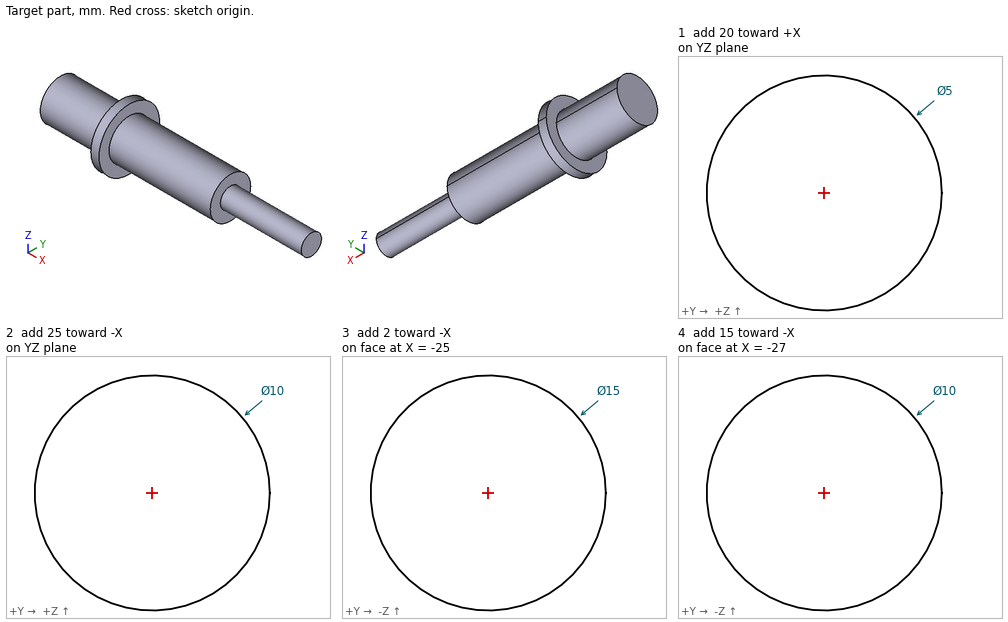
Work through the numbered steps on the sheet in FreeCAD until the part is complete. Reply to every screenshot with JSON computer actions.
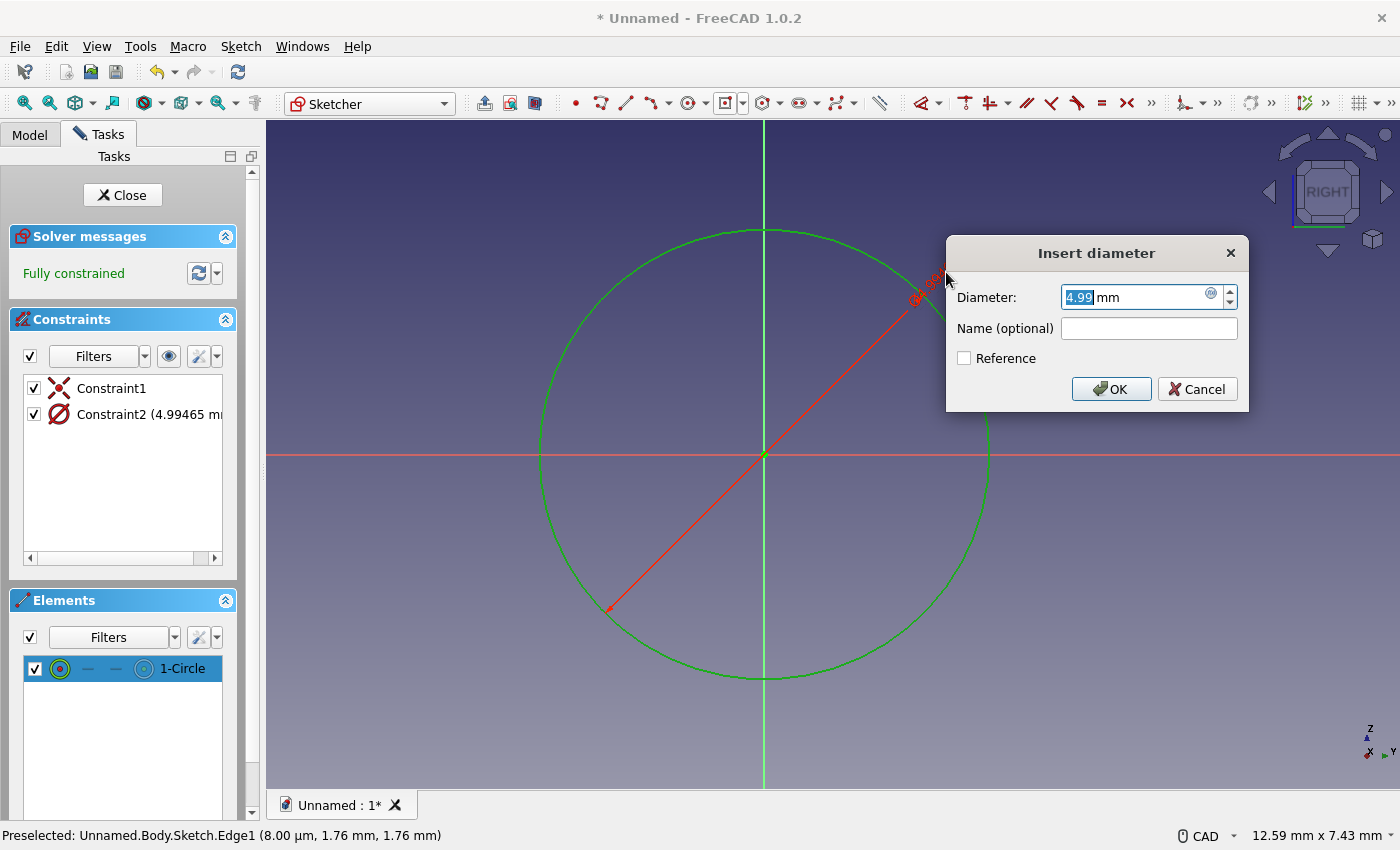
{"action": "type", "text": "5"}
{"action": "key", "text": "Return"}
{"action": "key", "text": "Escape"}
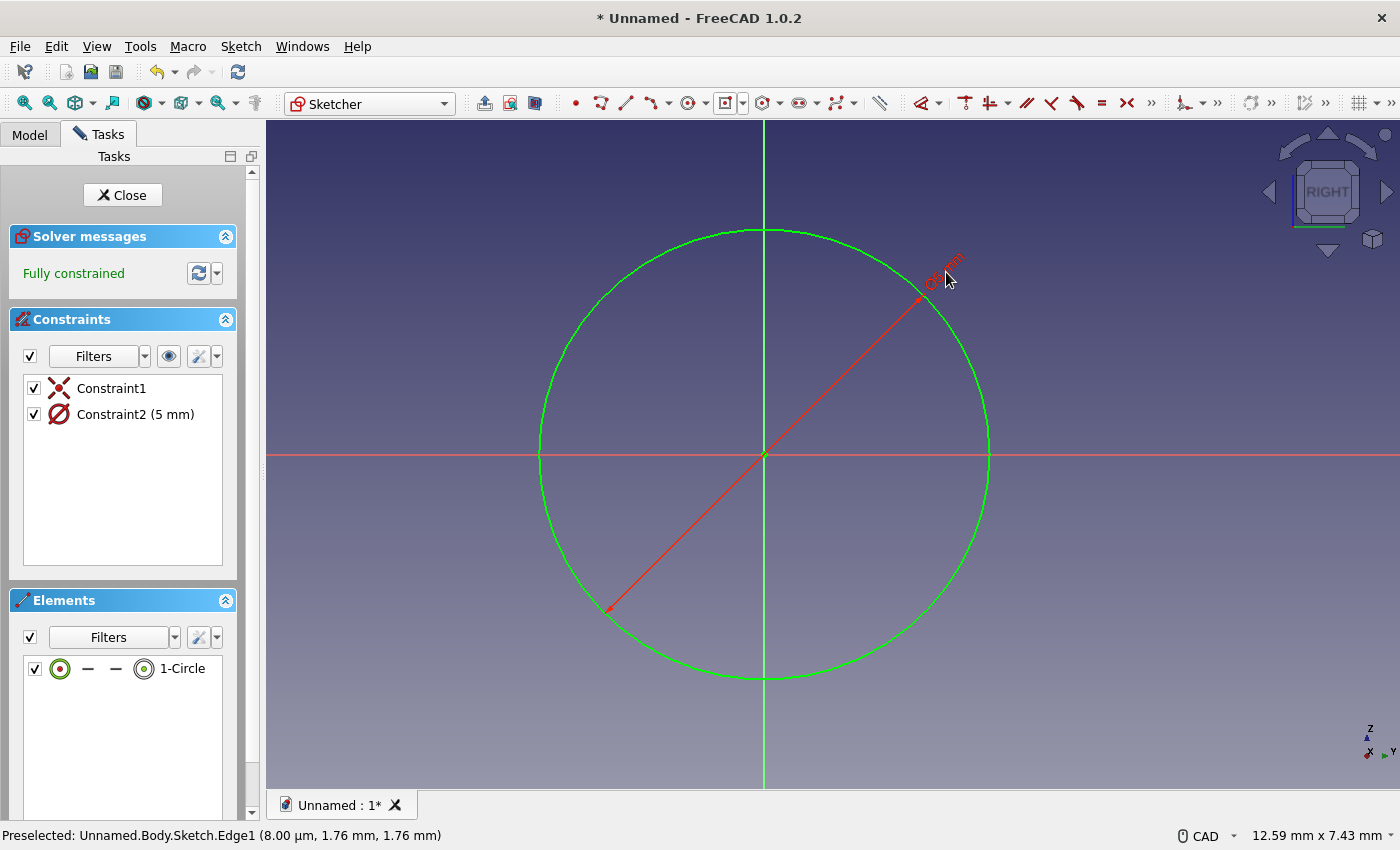
{"action": "left_click", "coordinate": [123, 195]}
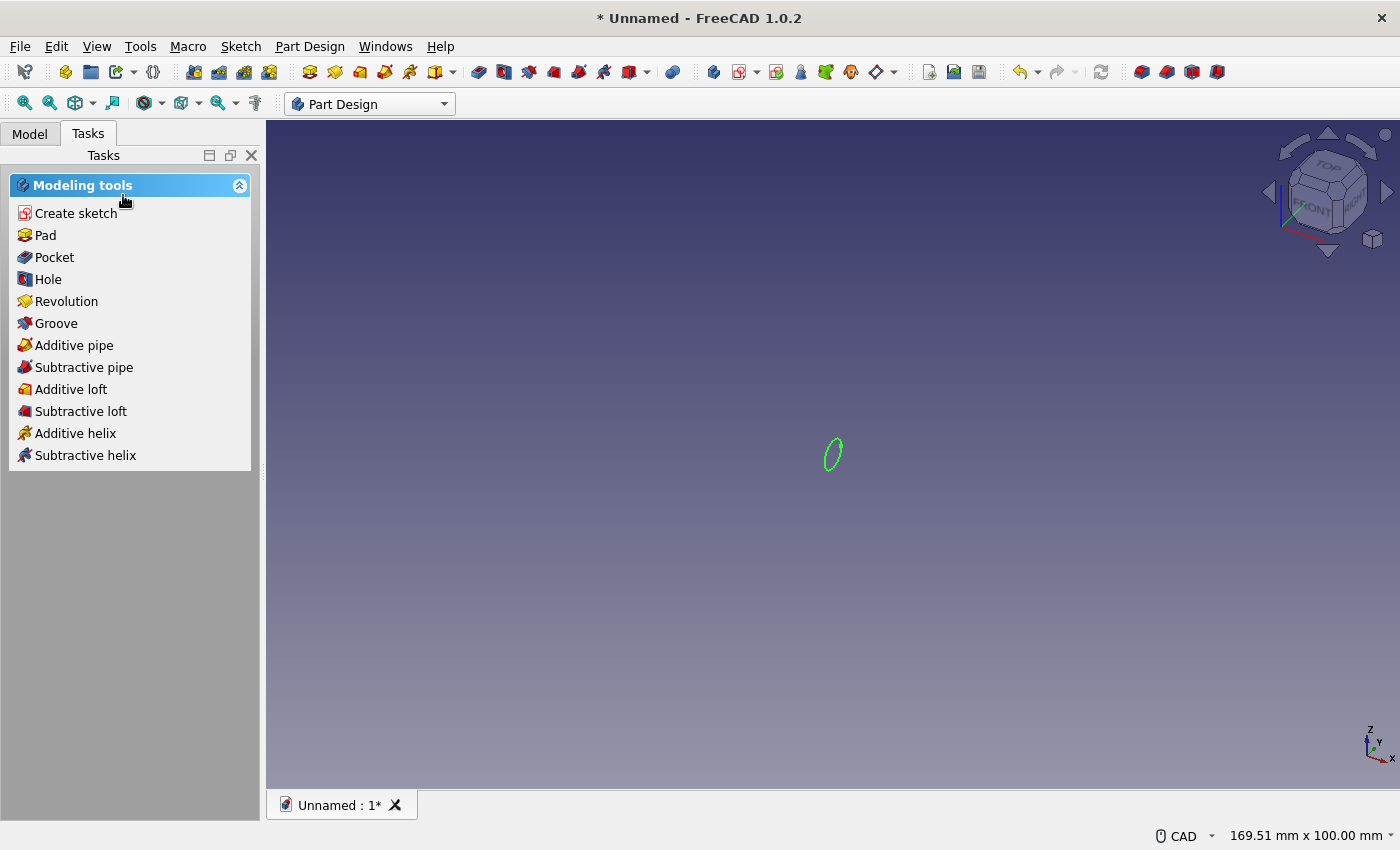
{"action": "left_click", "coordinate": [310, 72]}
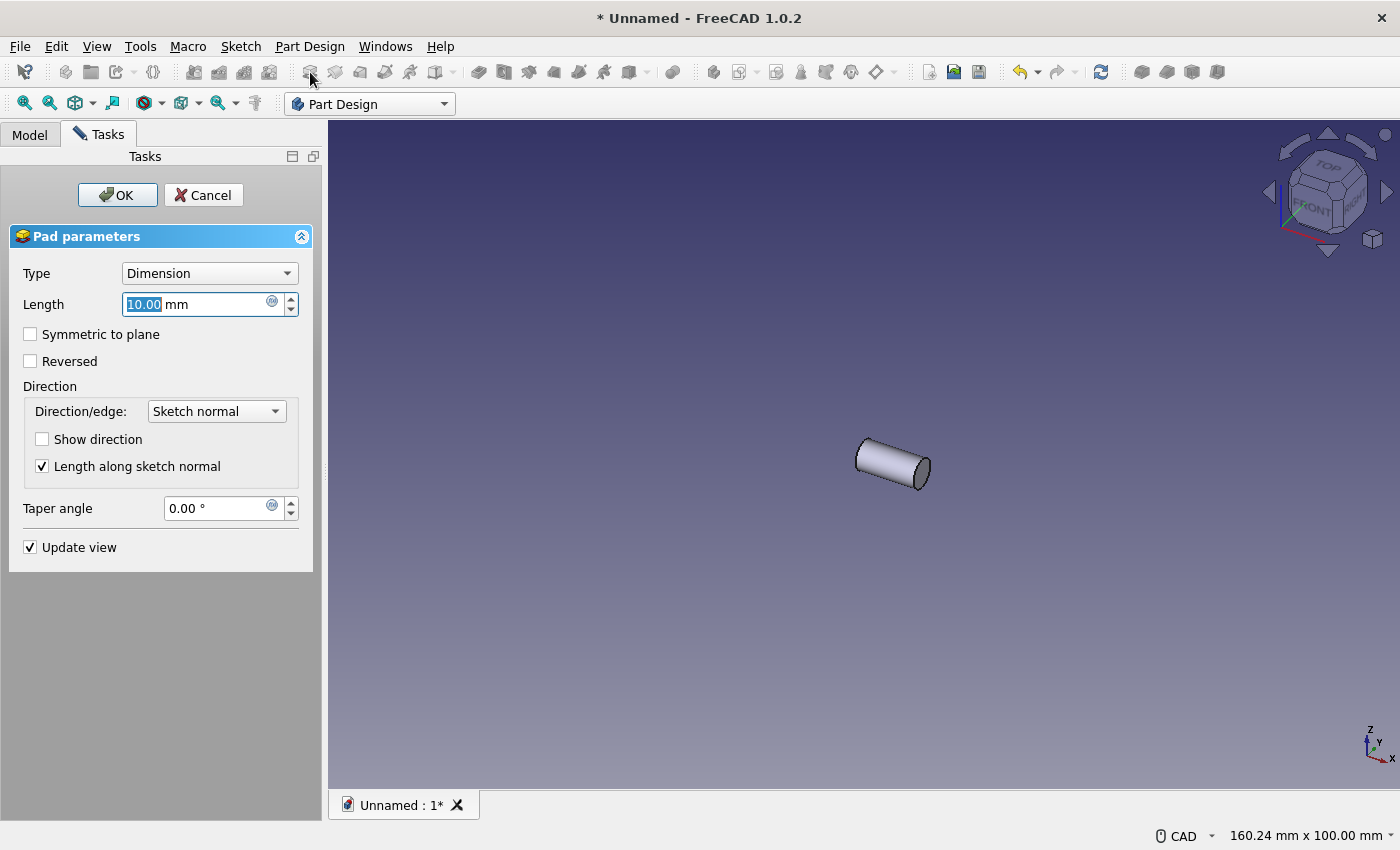
{"action": "type", "text": "20"}
{"action": "key", "text": "Tab"}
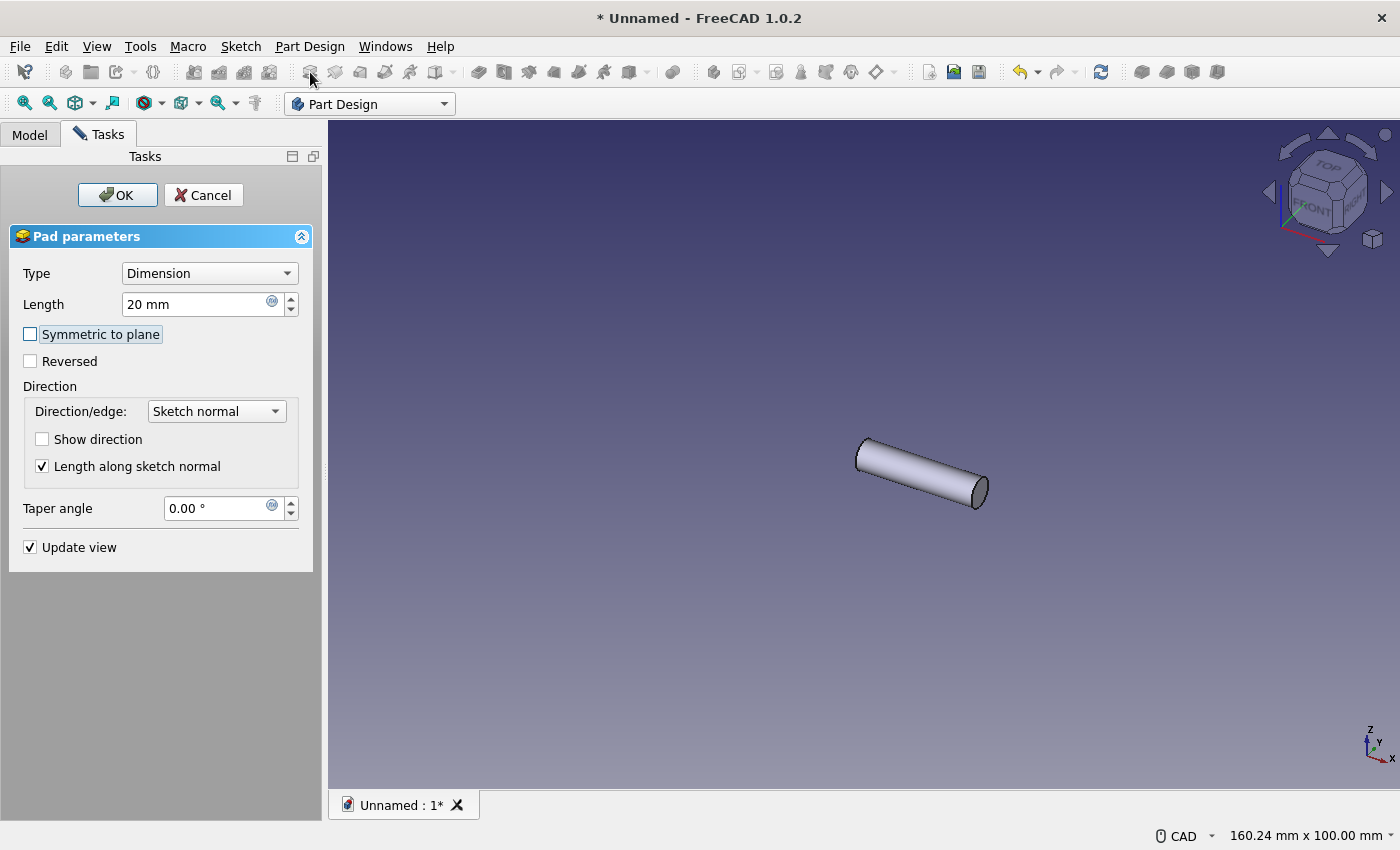
{"action": "left_click", "coordinate": [118, 195]}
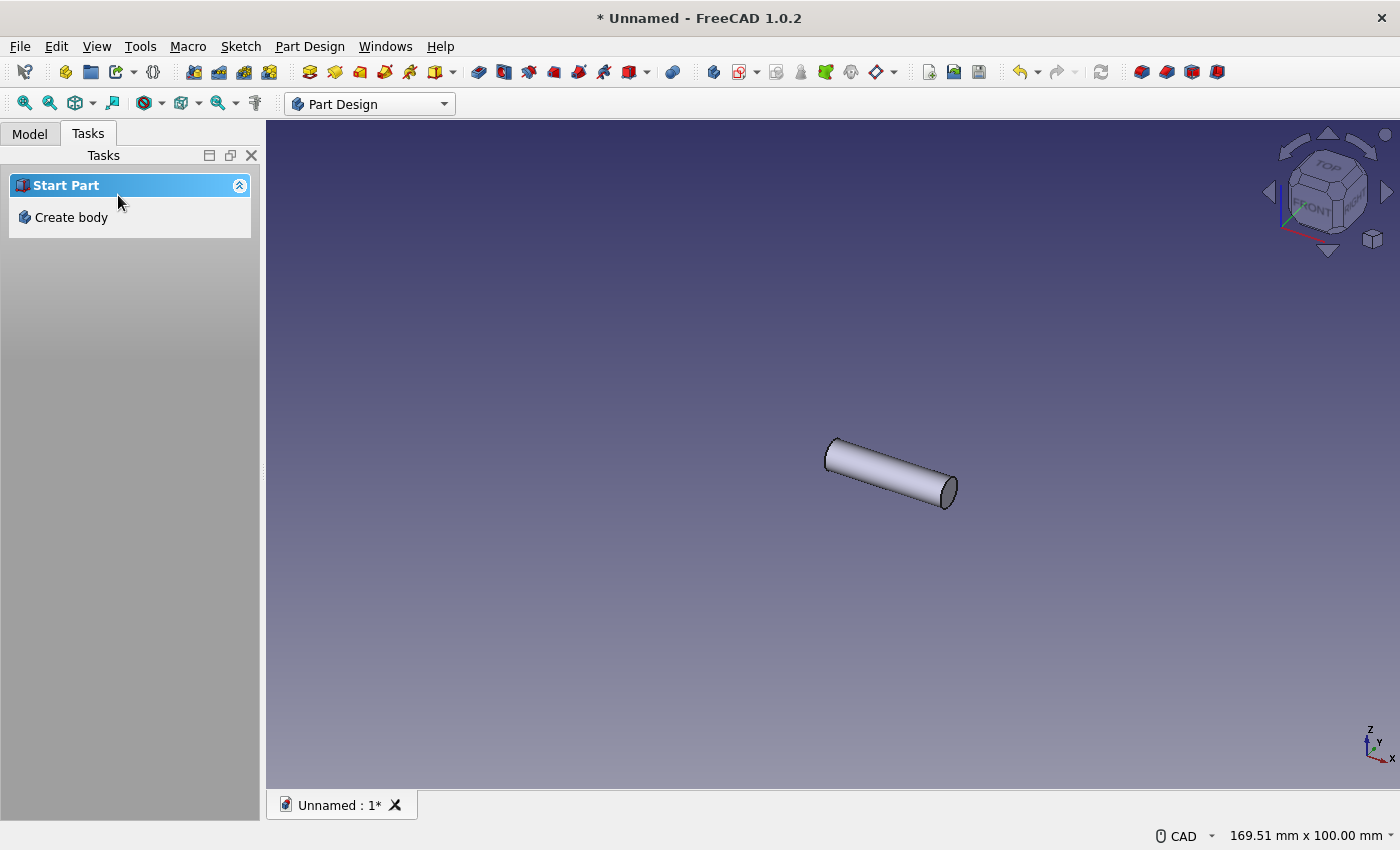
{"action": "key", "text": "v f"}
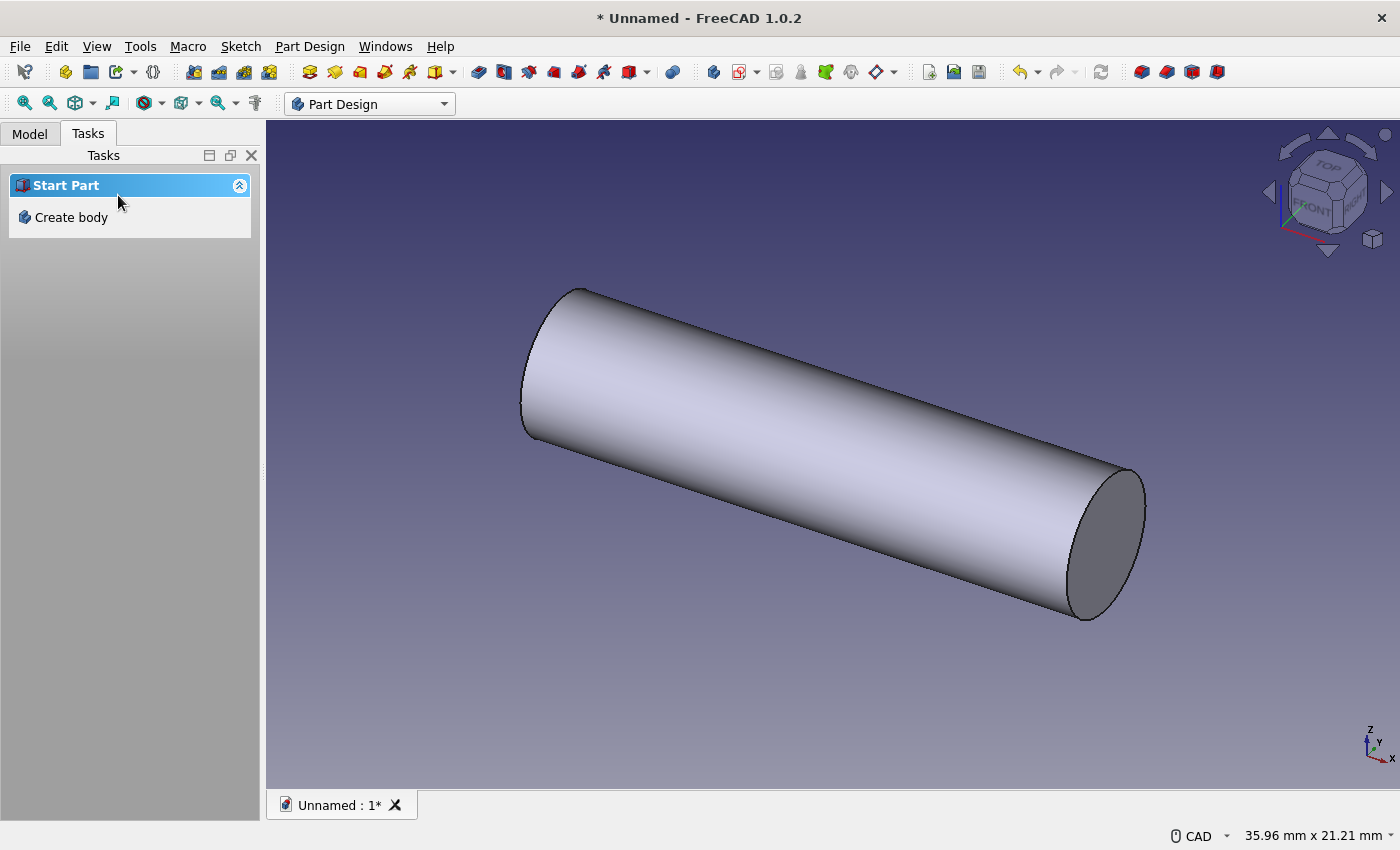
{"action": "left_click", "coordinate": [738, 72]}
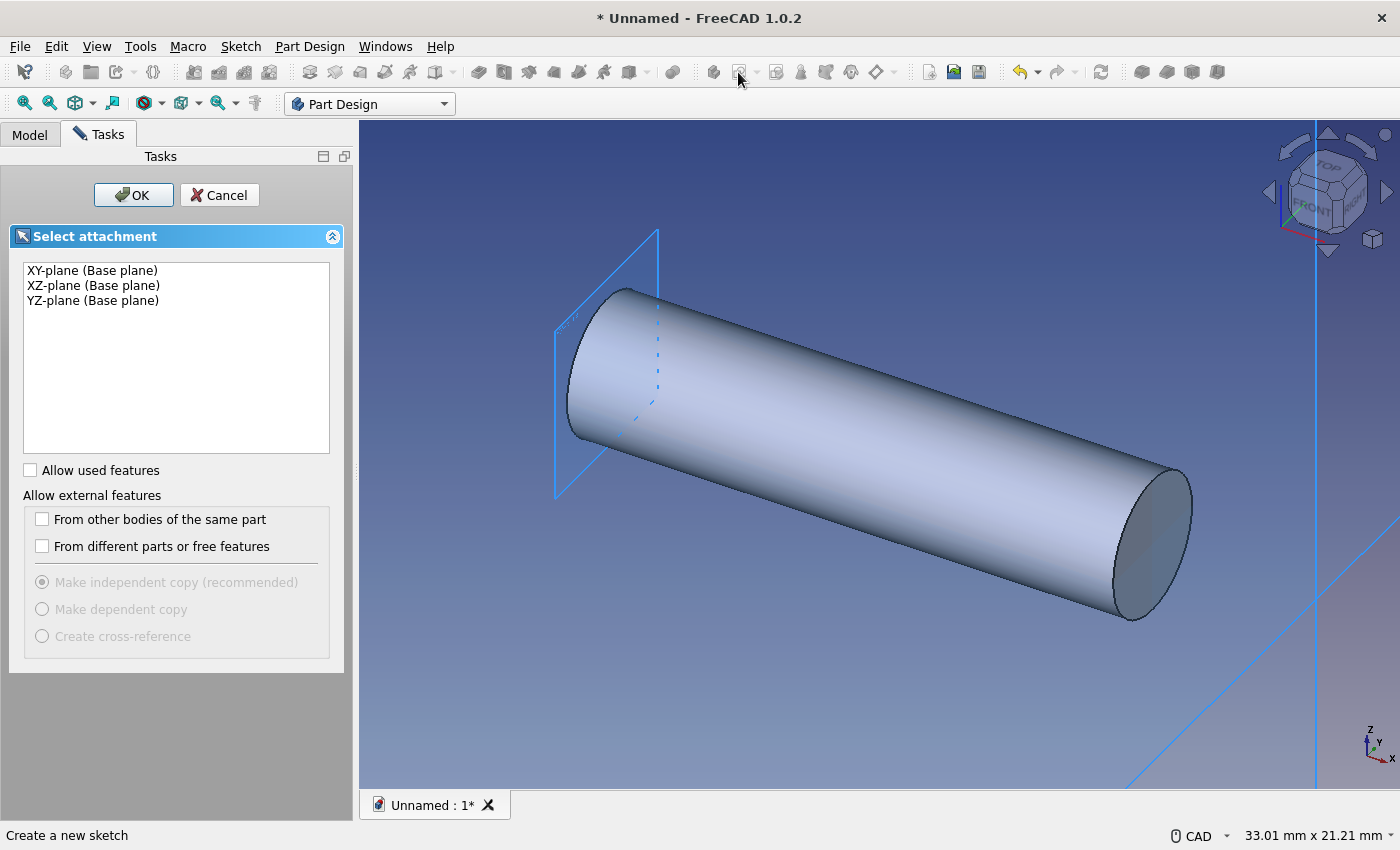
{"action": "left_click", "coordinate": [84, 300]}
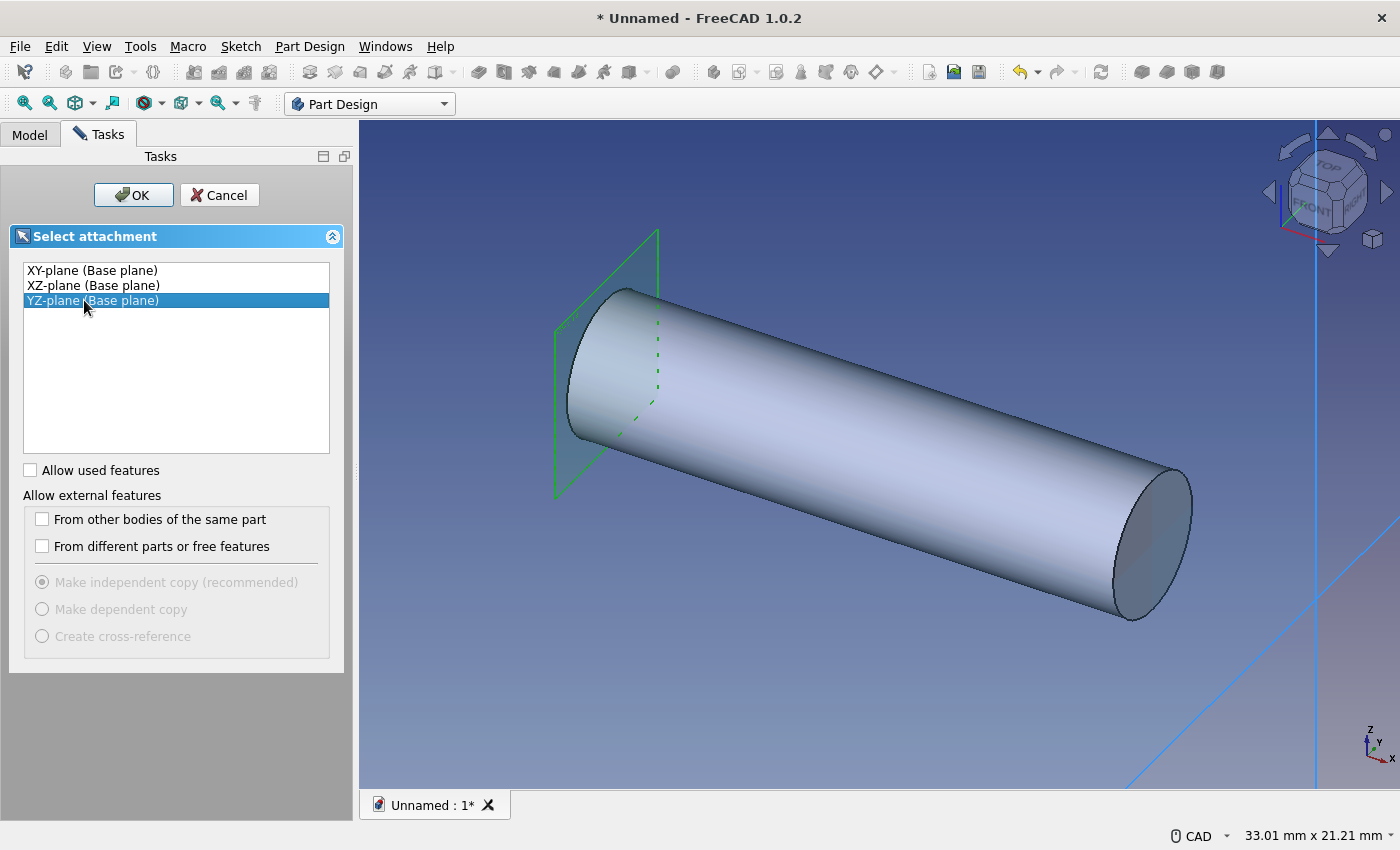
{"action": "left_click", "coordinate": [134, 195]}